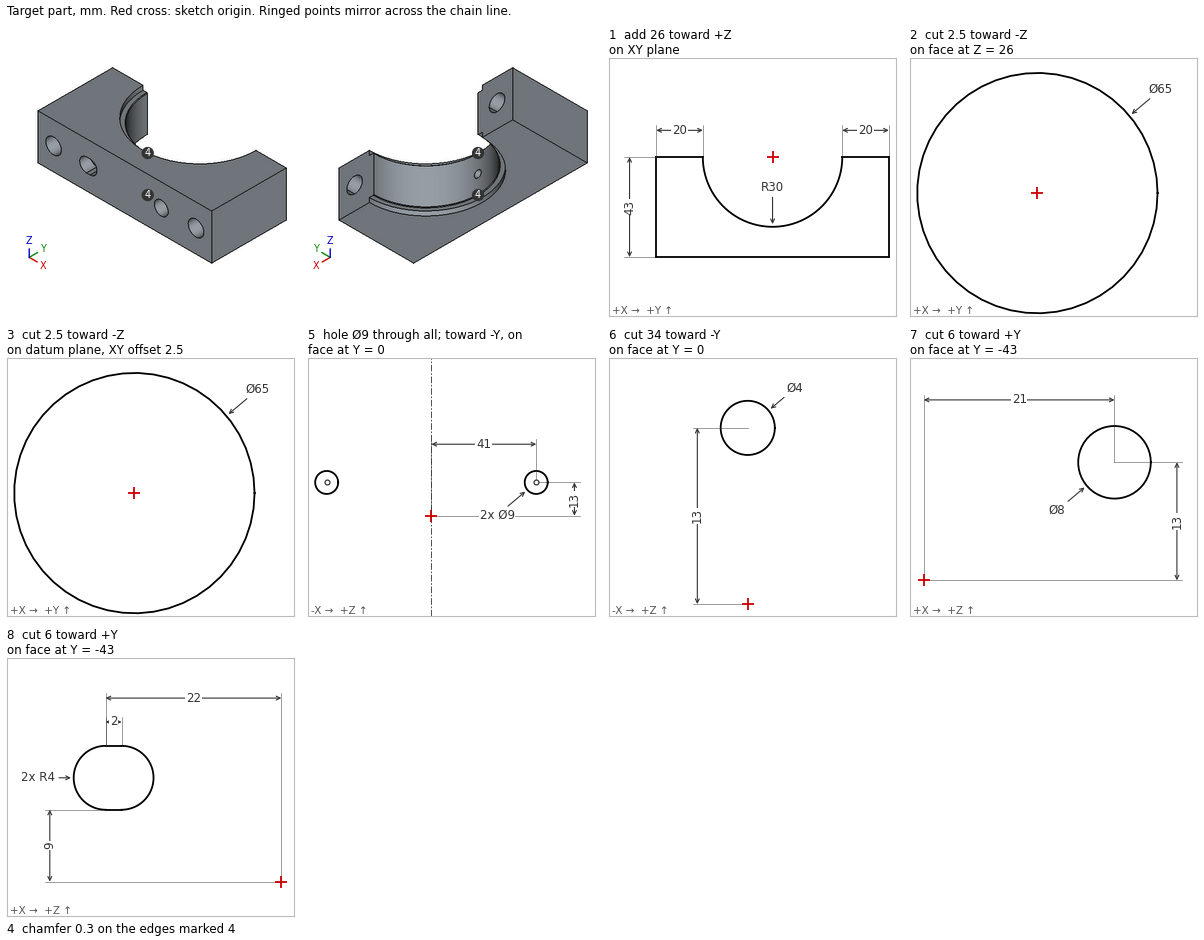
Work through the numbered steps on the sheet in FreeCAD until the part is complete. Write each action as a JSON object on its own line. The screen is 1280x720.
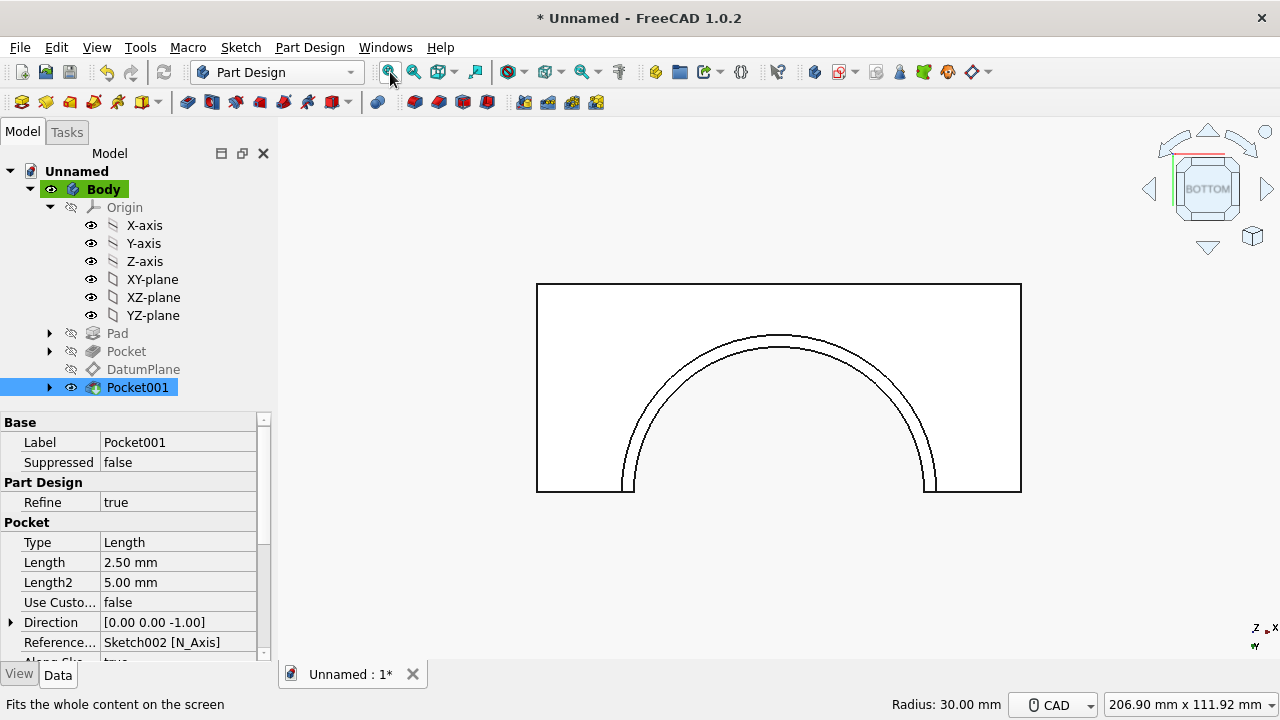
{"action": "left_click", "coordinate": [779, 346], "text": "ctrl"}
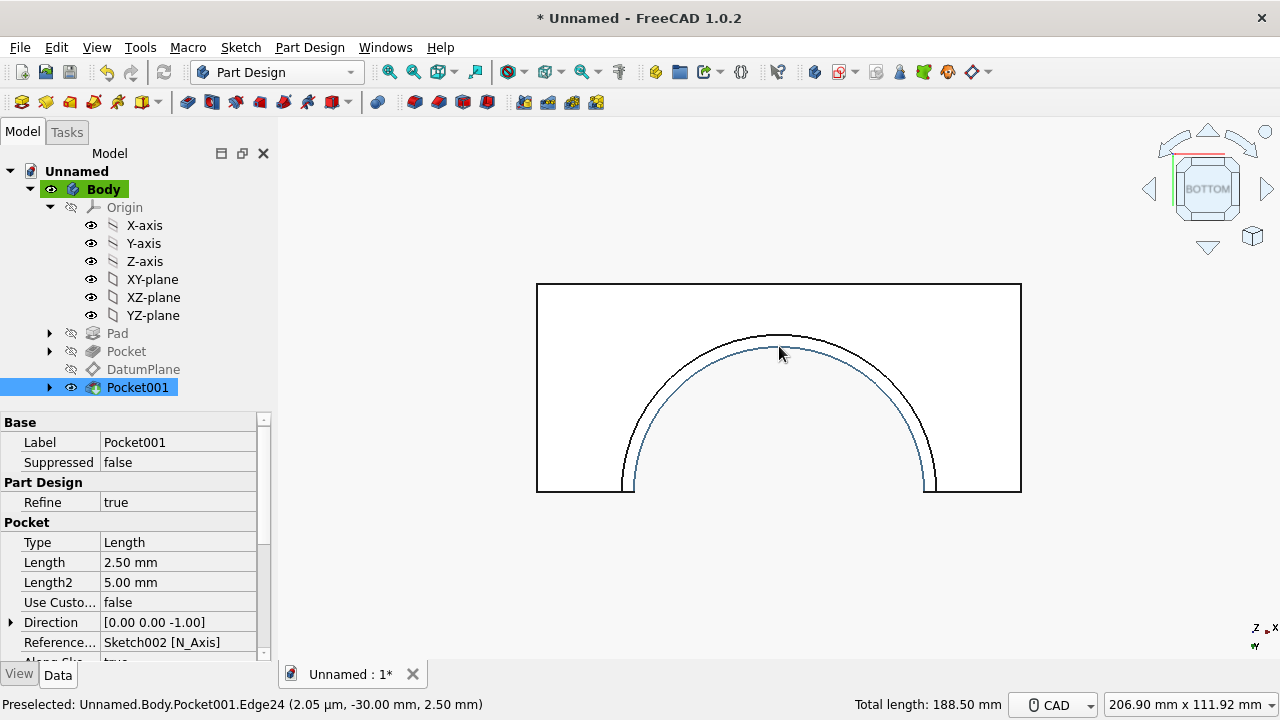
{"action": "left_click", "coordinate": [440, 102]}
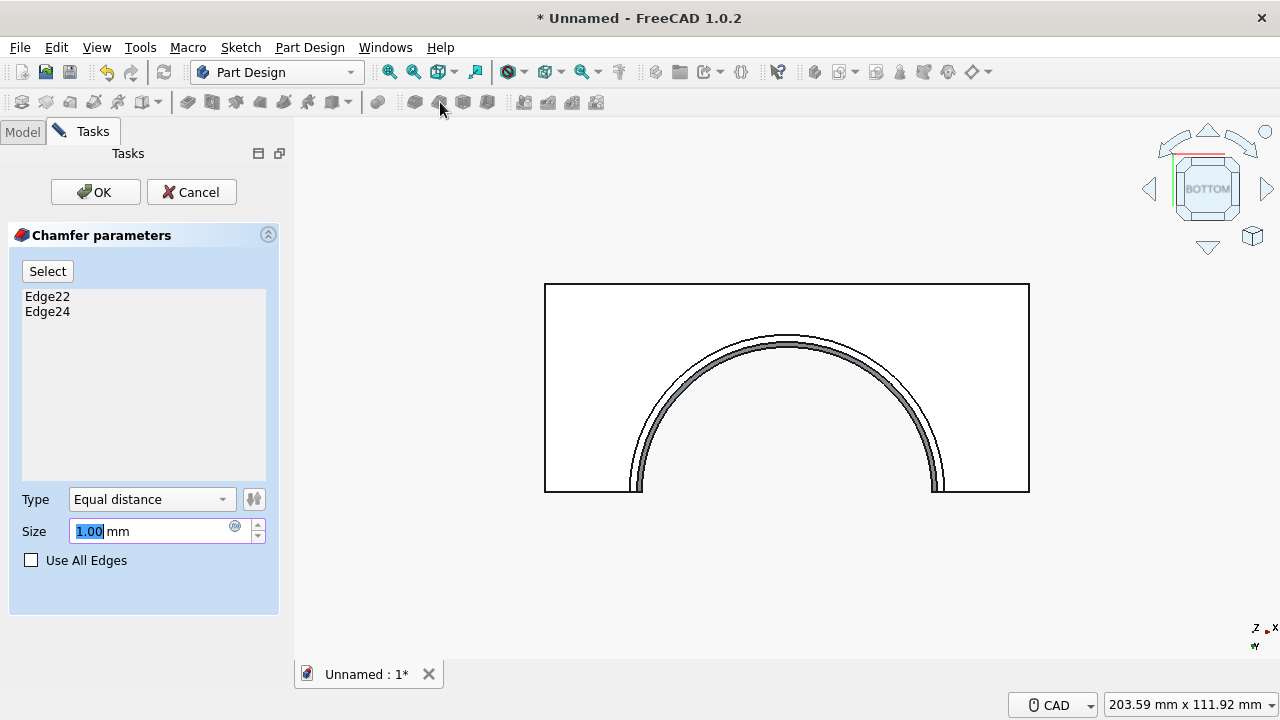
{"action": "type", "text": "0.3"}
{"action": "key", "text": "Tab"}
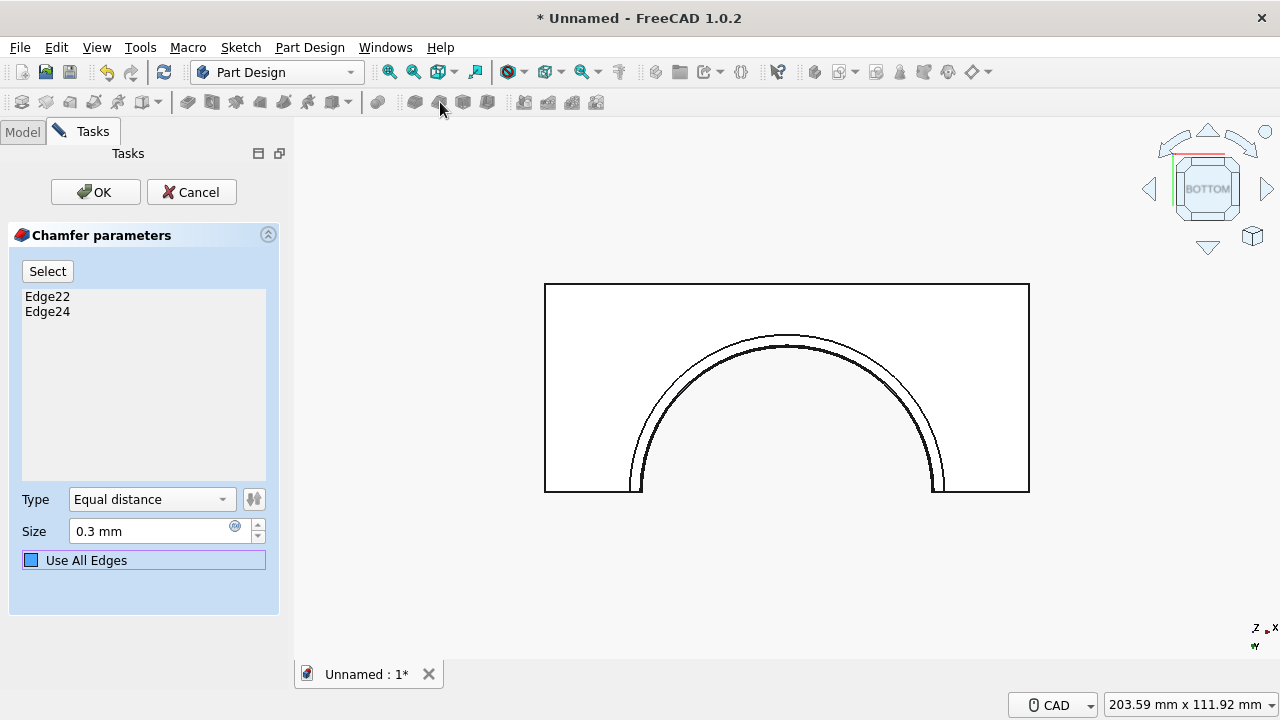
{"action": "left_click", "coordinate": [96, 192]}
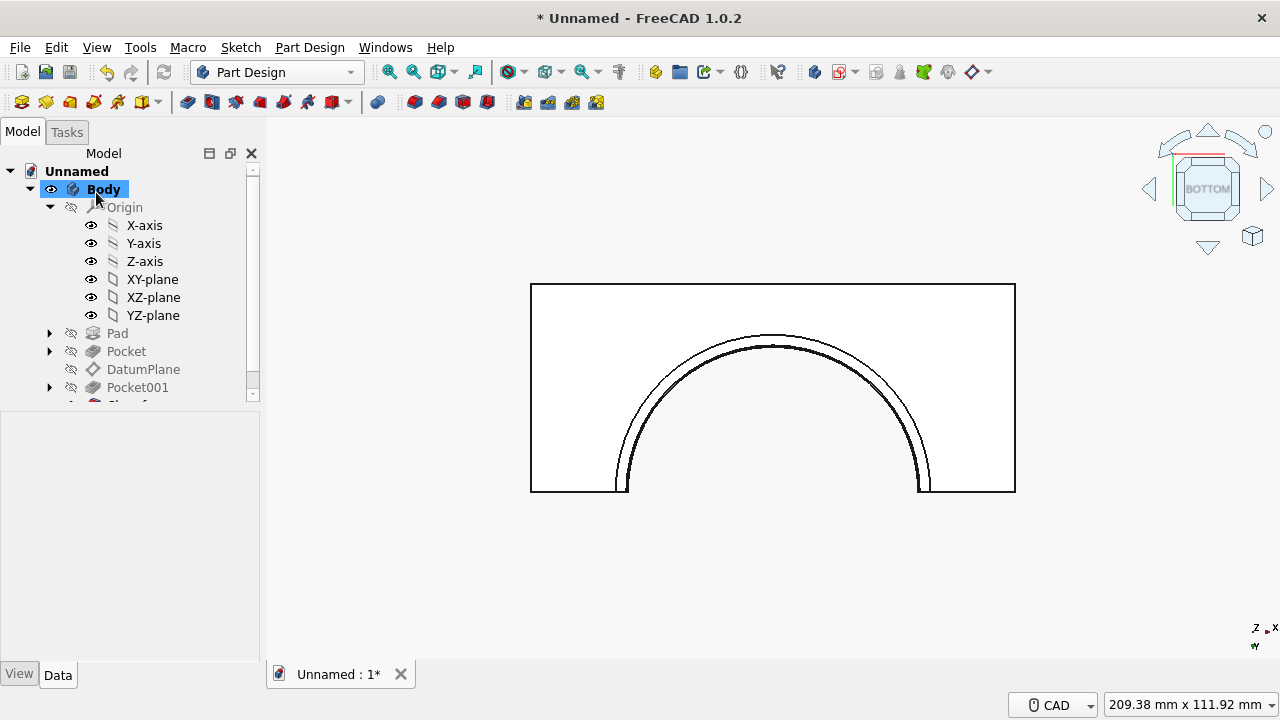
{"action": "key", "text": "4"}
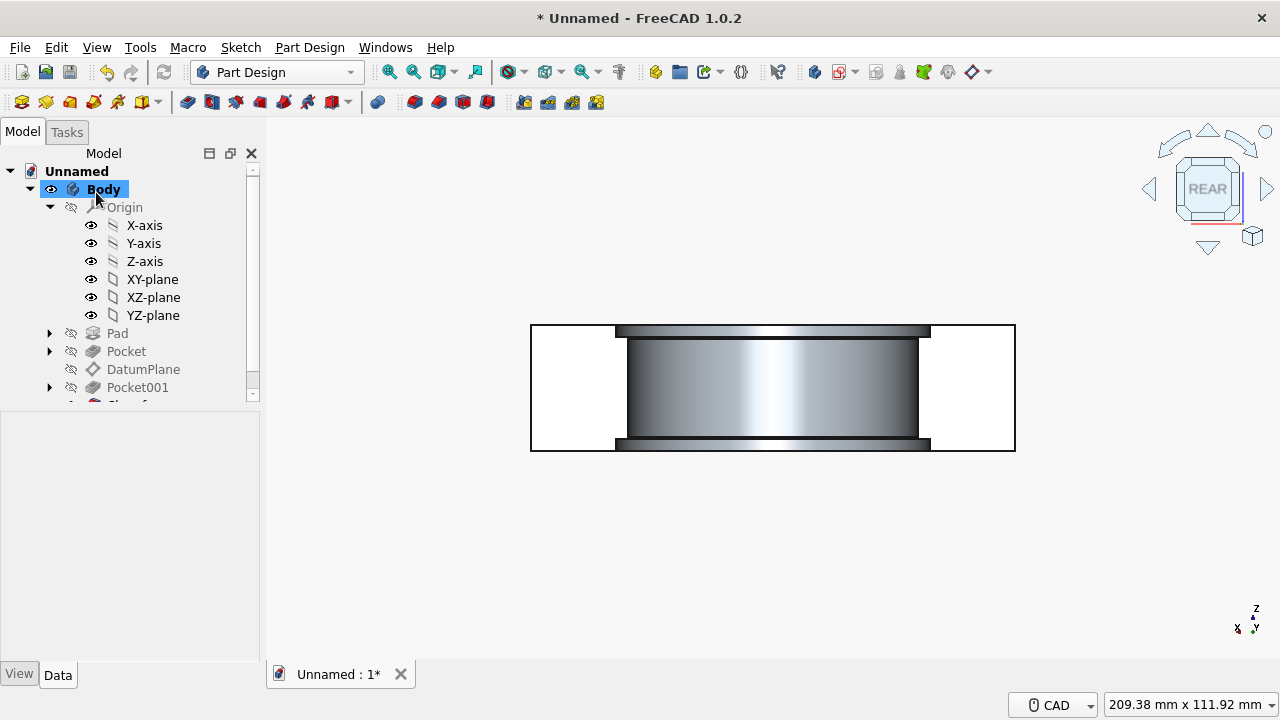
{"action": "left_click", "coordinate": [967, 387]}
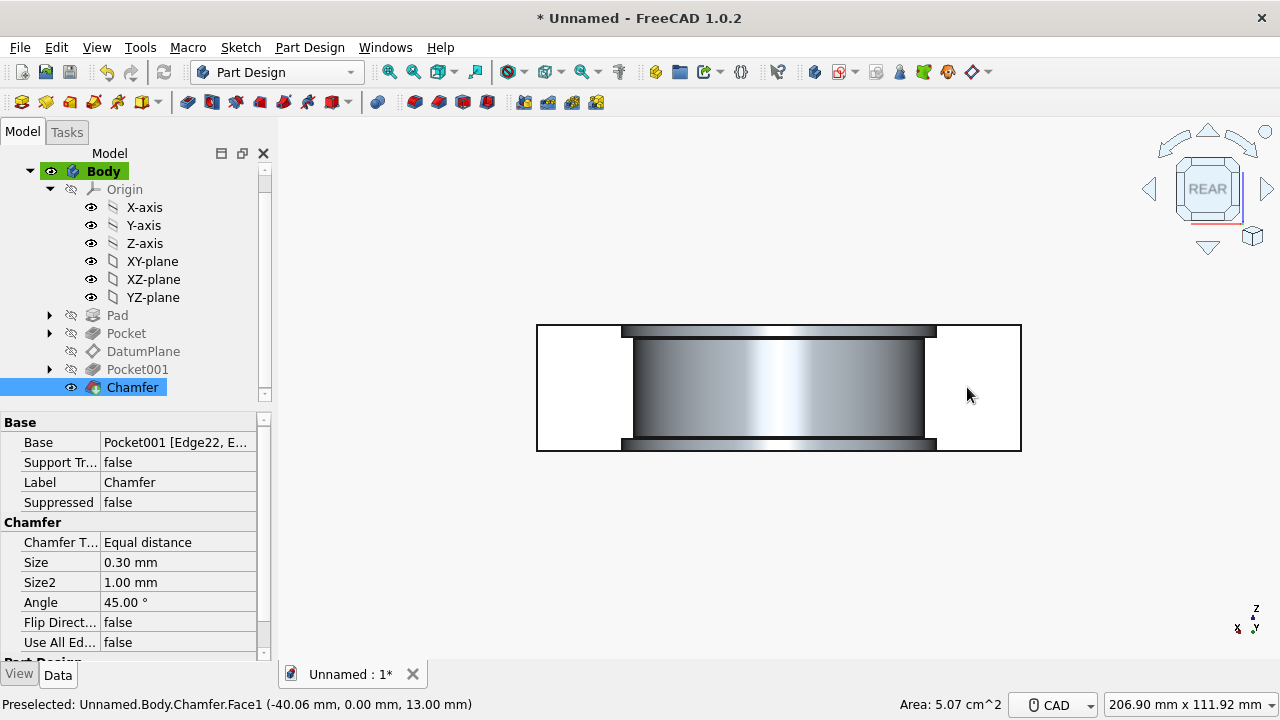
{"action": "left_click", "coordinate": [840, 72]}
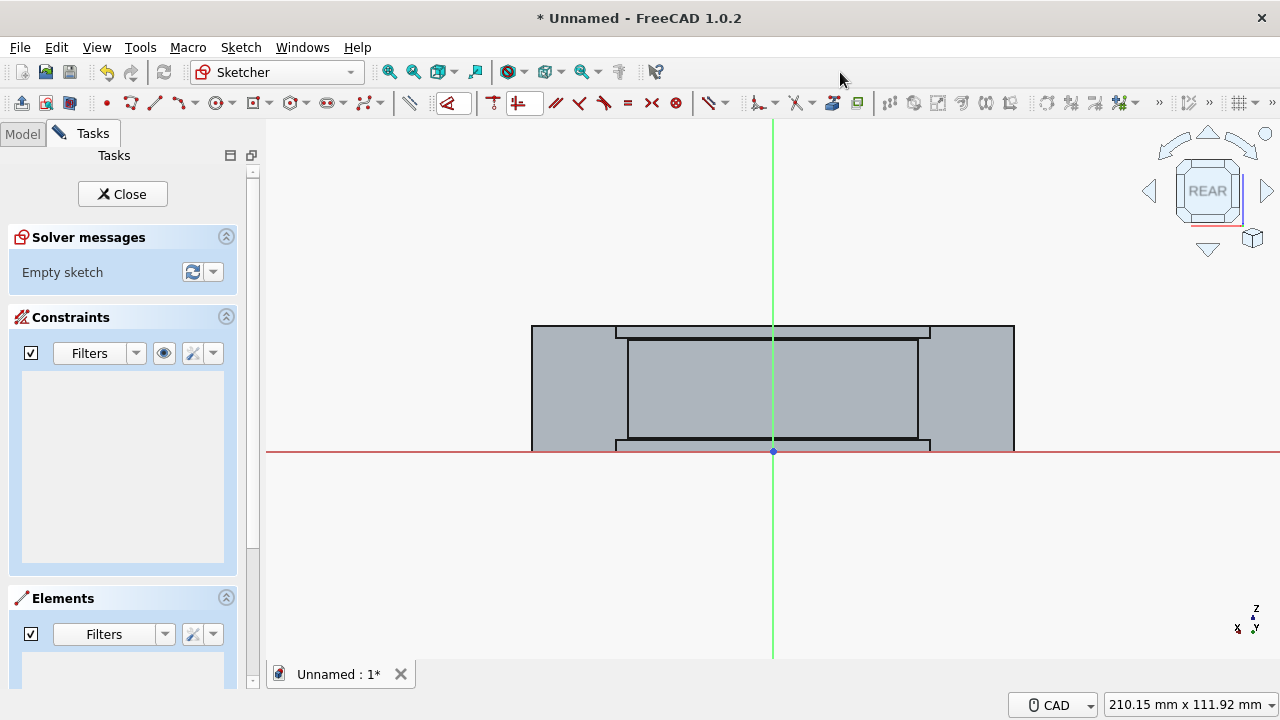
{"action": "left_click", "coordinate": [216, 104]}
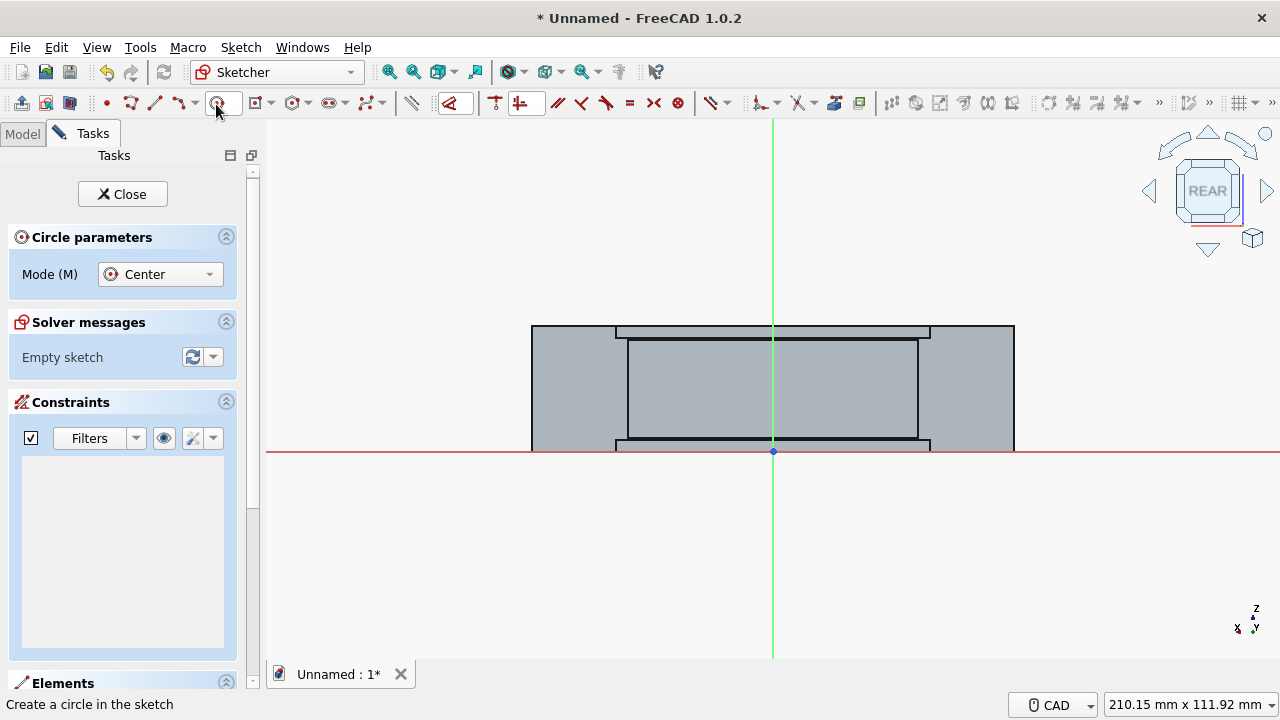
{"action": "left_click", "coordinate": [971, 389]}
{"action": "left_click", "coordinate": [986, 374]}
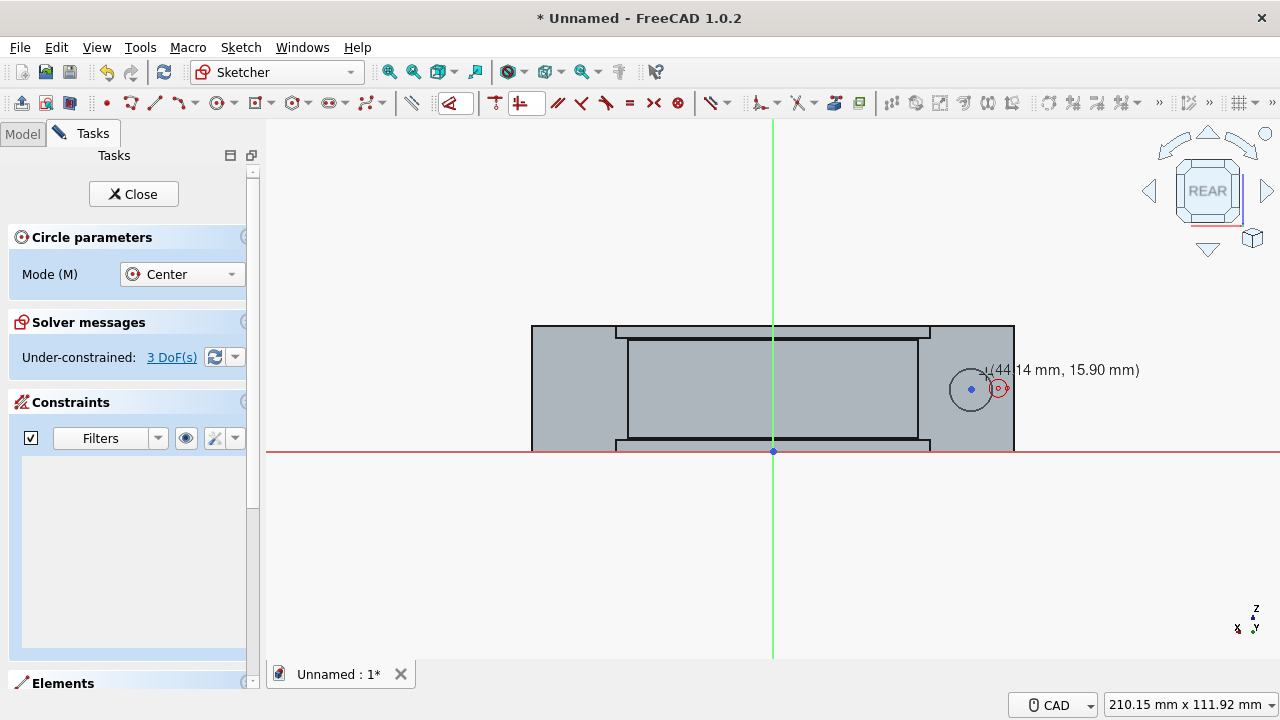
{"action": "left_click", "coordinate": [575, 389]}
{"action": "left_click", "coordinate": [591, 374]}
{"action": "key", "text": "Escape"}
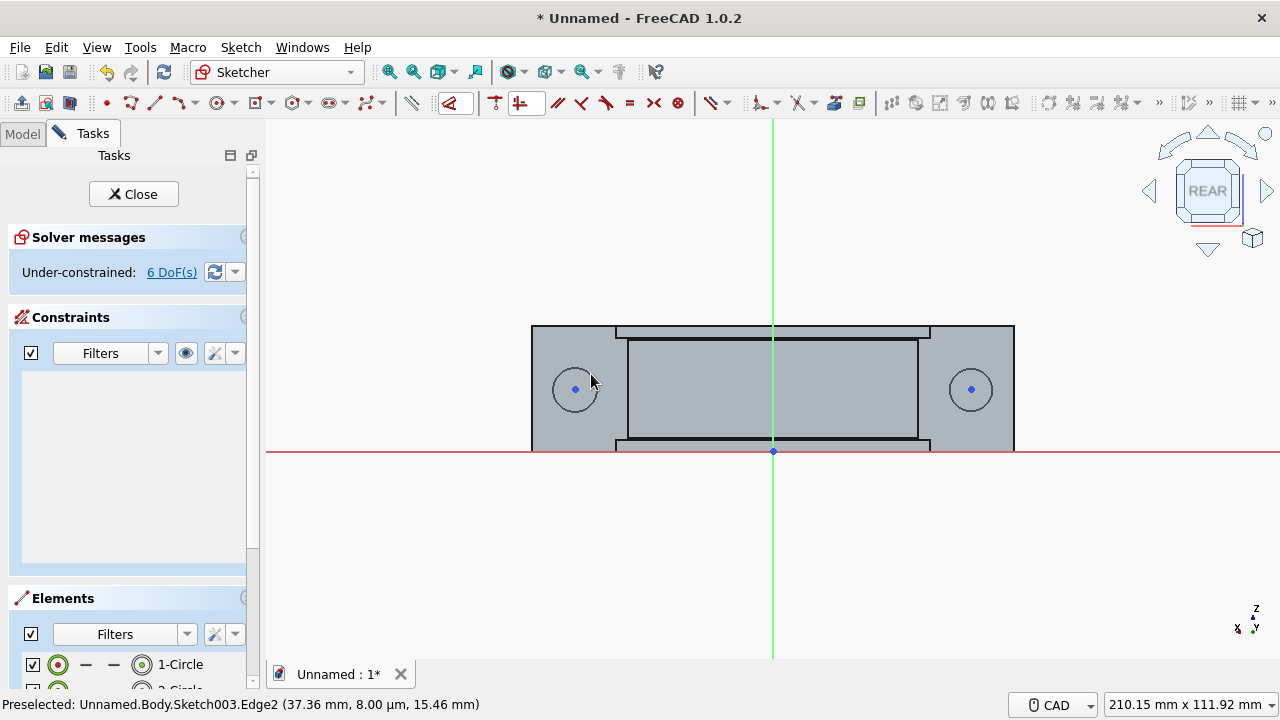
{"action": "left_click", "coordinate": [986, 375]}